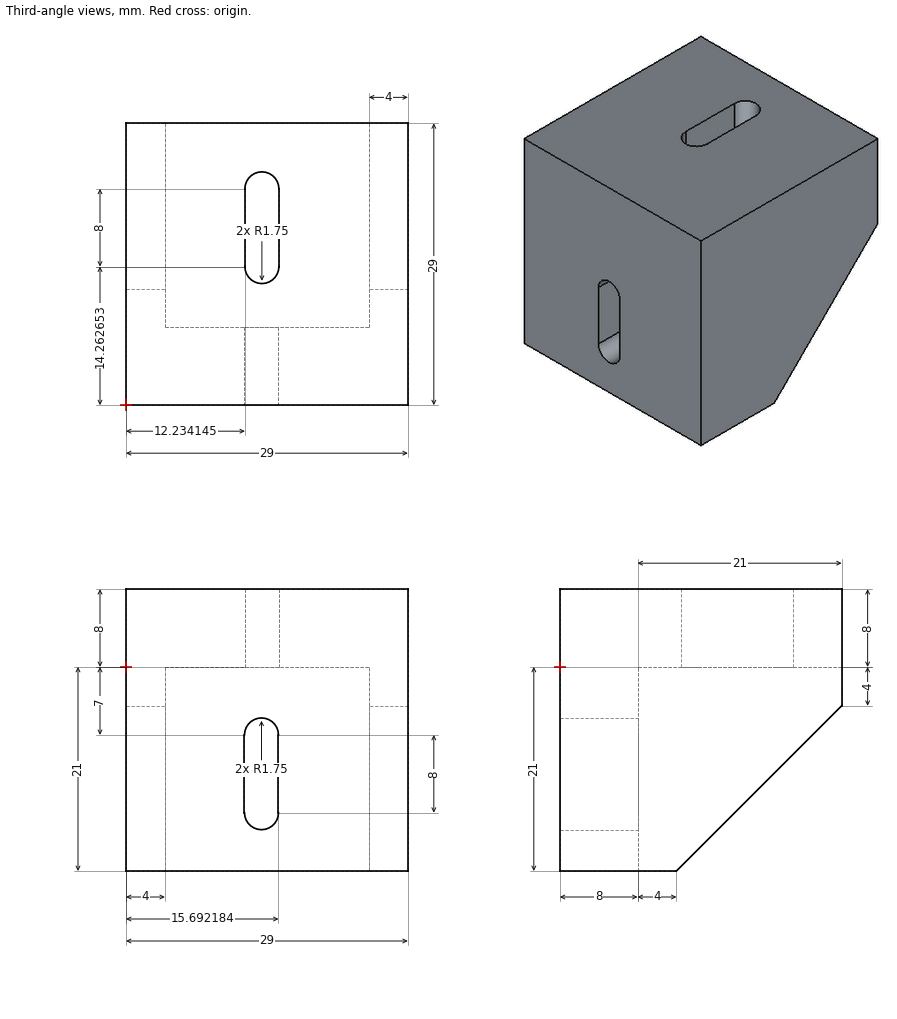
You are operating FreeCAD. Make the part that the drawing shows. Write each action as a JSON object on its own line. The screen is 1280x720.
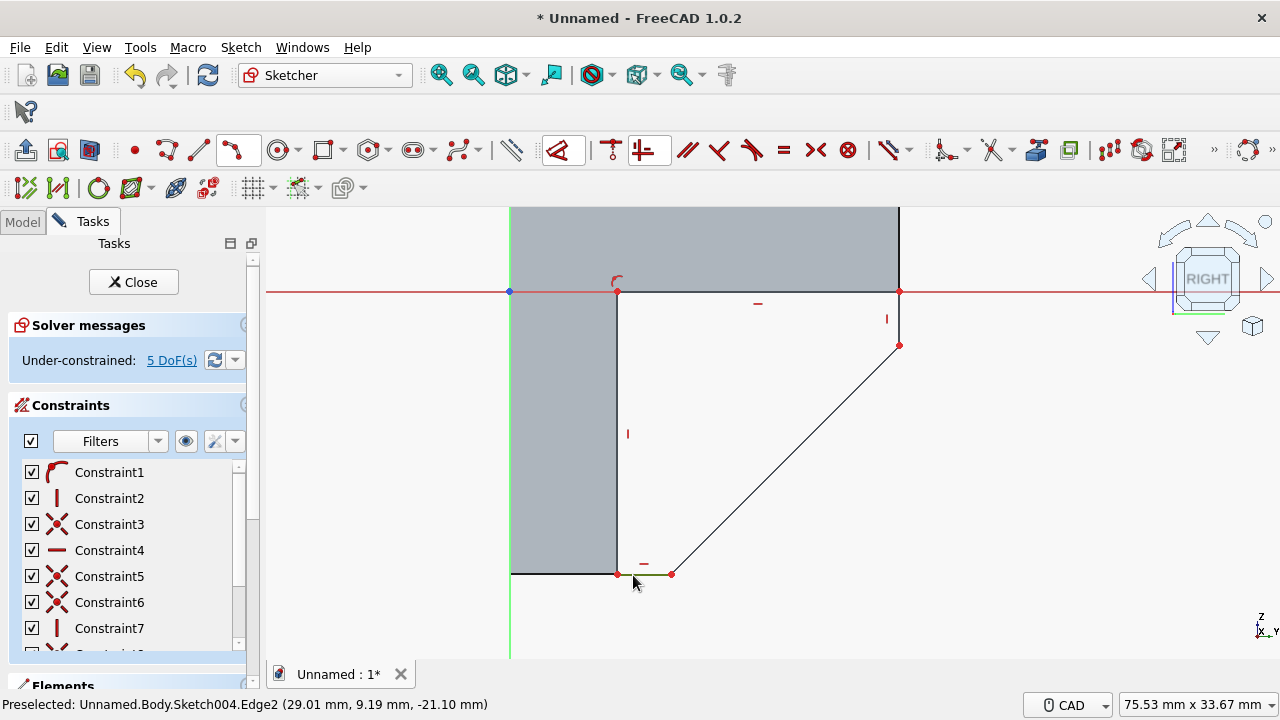
{"action": "left_click", "coordinate": [580, 150]}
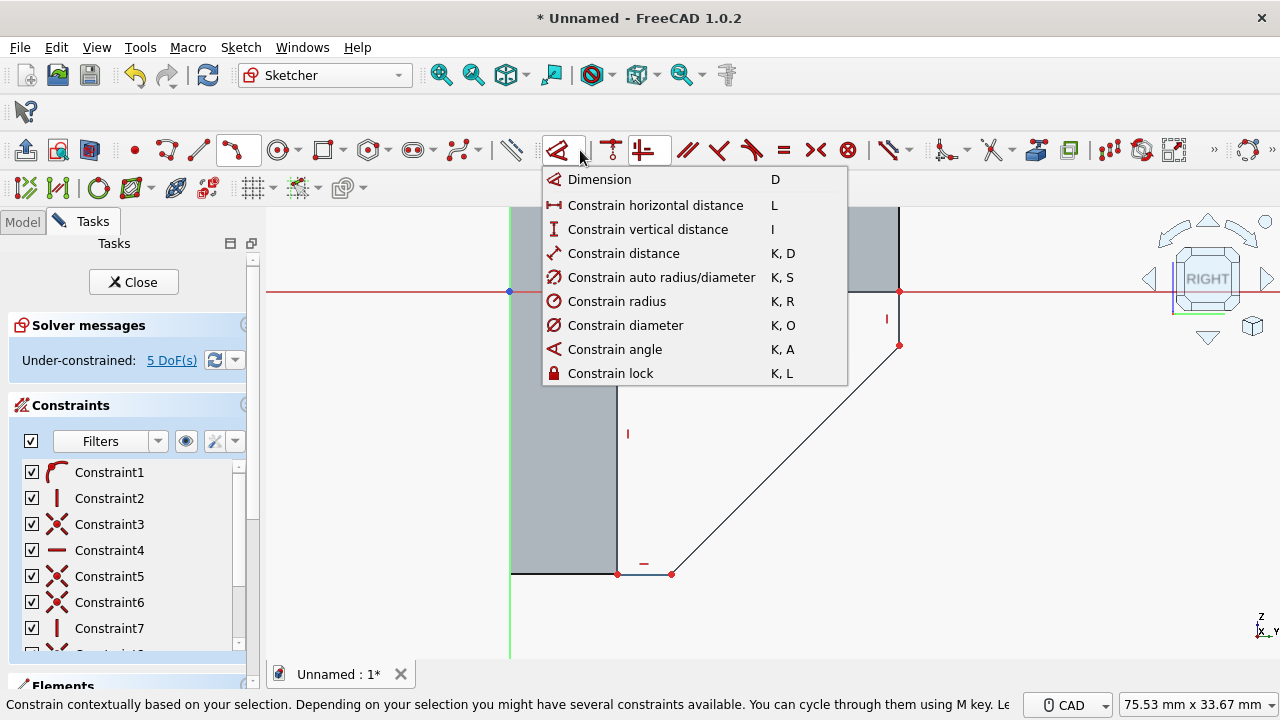
{"action": "left_click", "coordinate": [695, 205]}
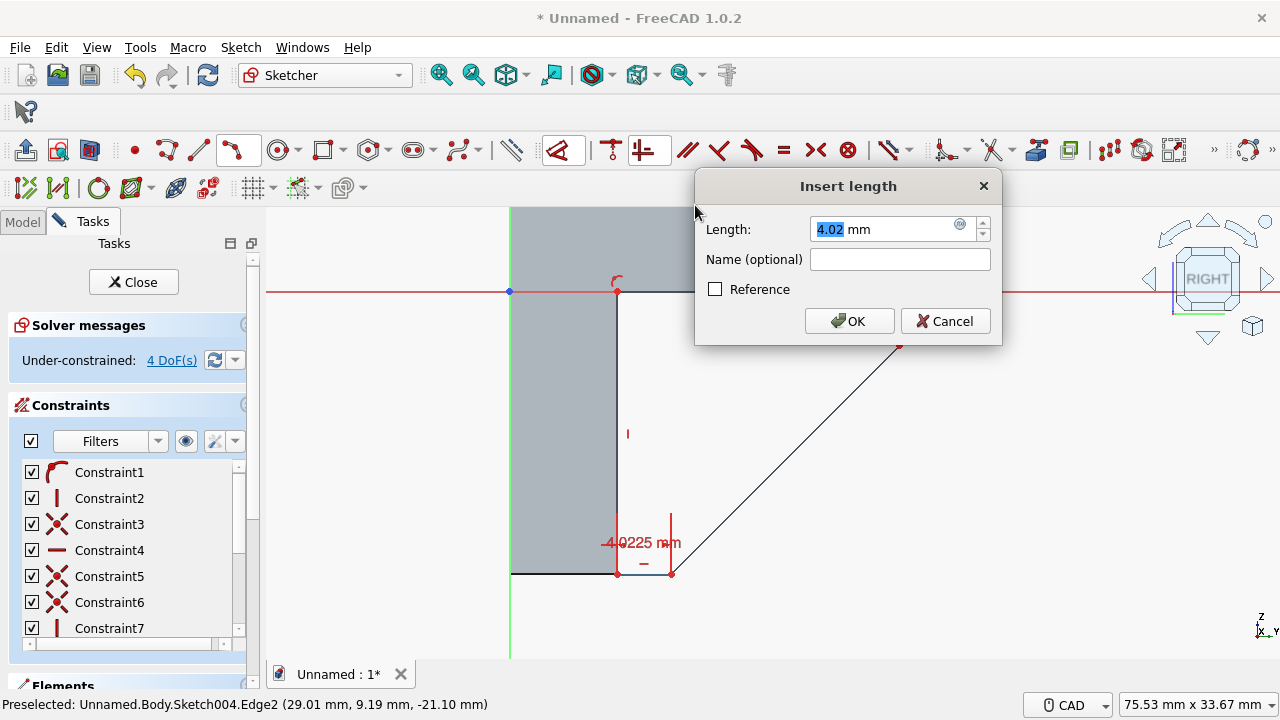
{"action": "type", "text": "4"}
{"action": "key", "text": "Return"}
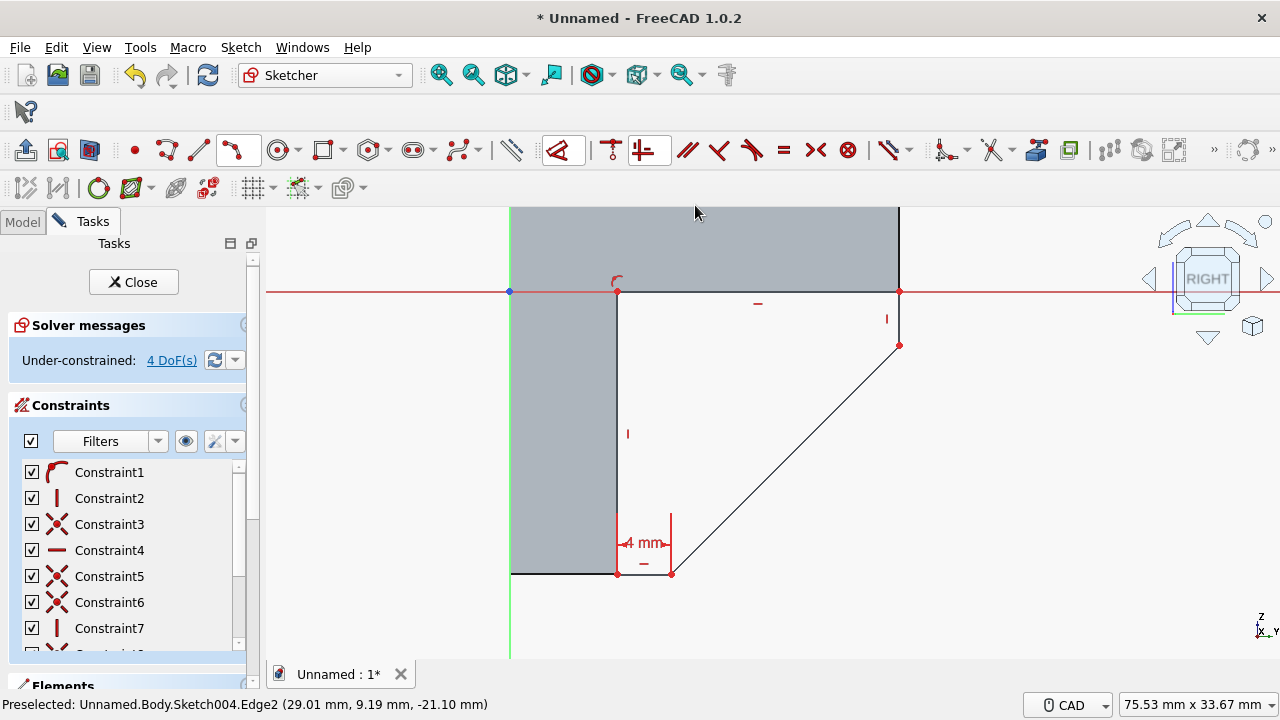
{"action": "left_click", "coordinate": [899, 330]}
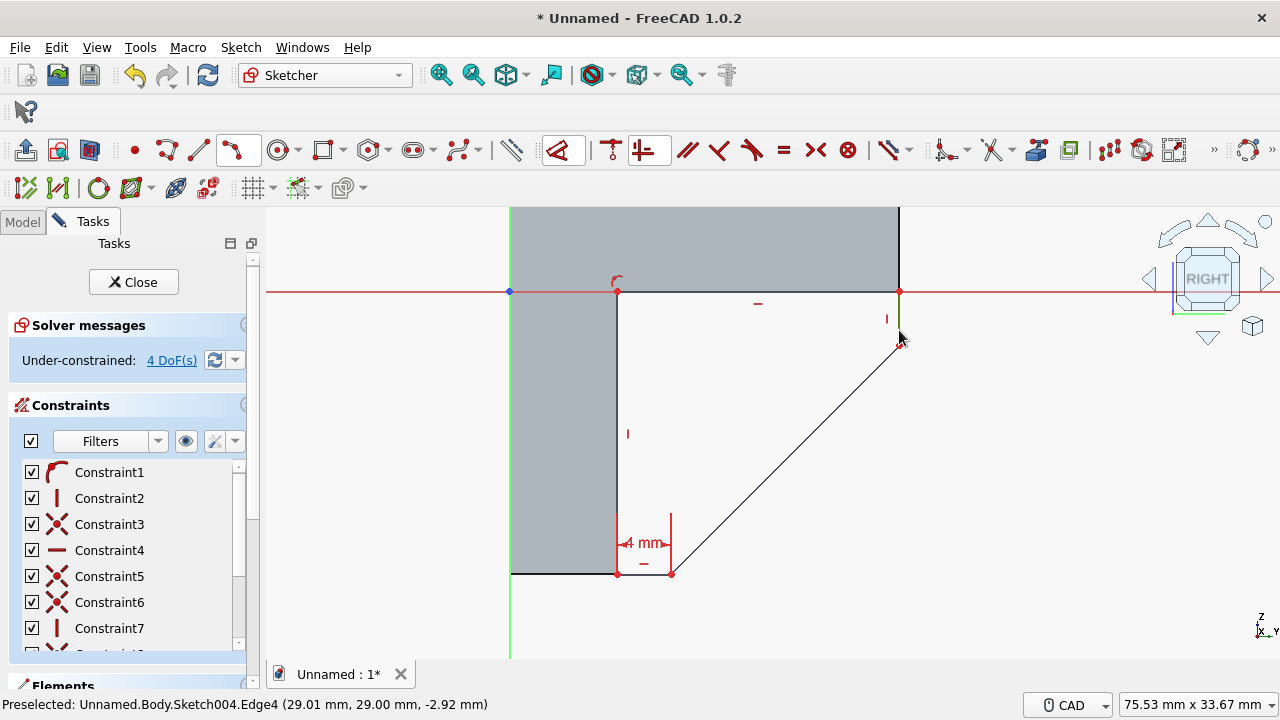
{"action": "key", "text": "i"}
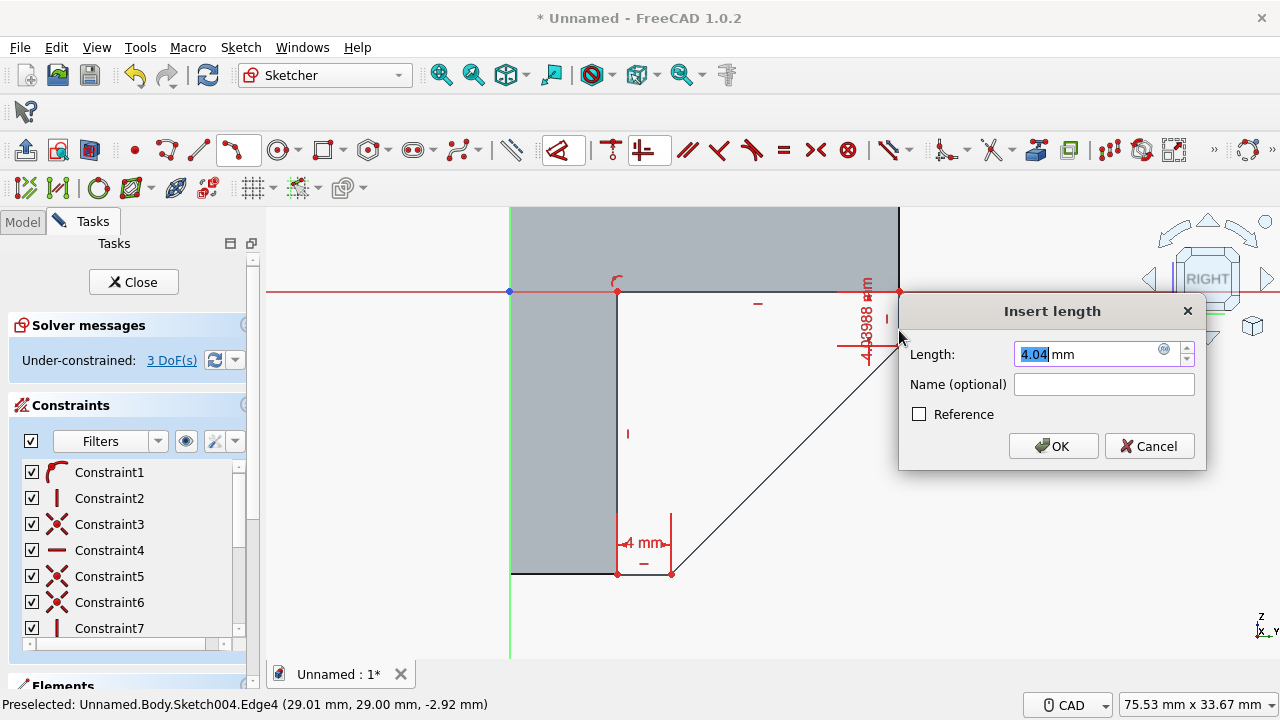
{"action": "type", "text": "4"}
{"action": "key", "text": "Return"}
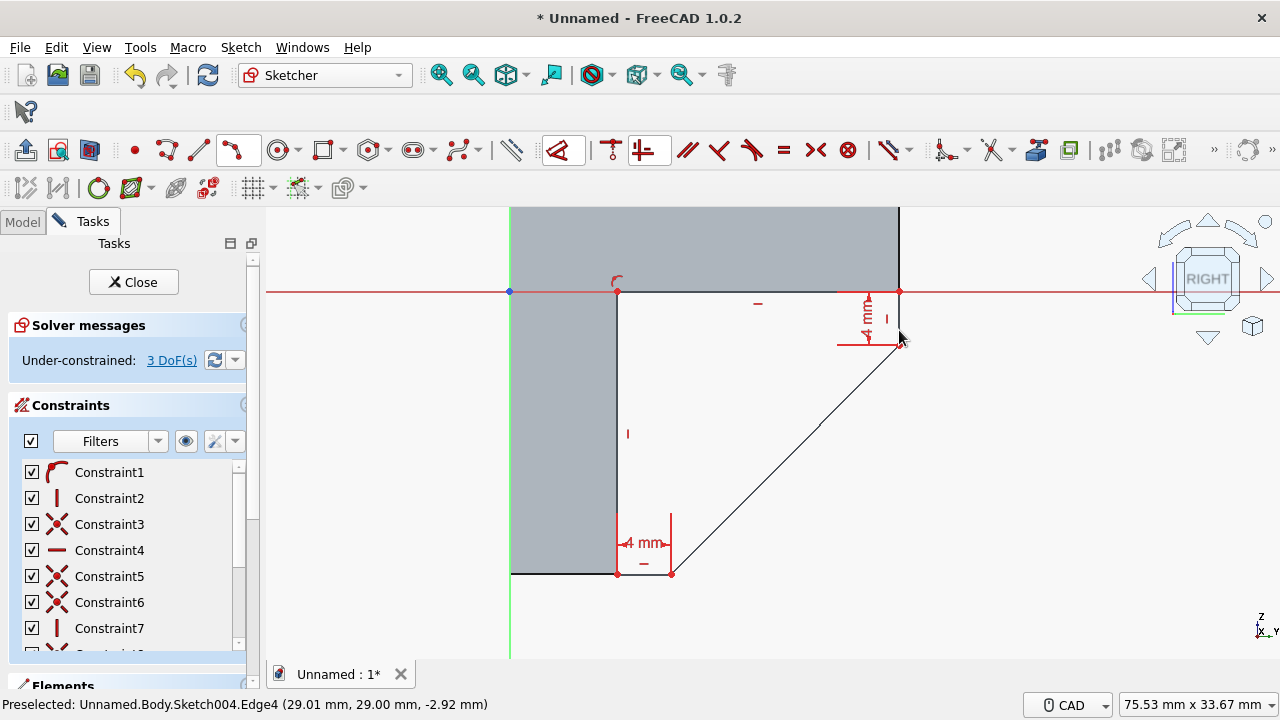
{"action": "left_click", "coordinate": [617, 377]}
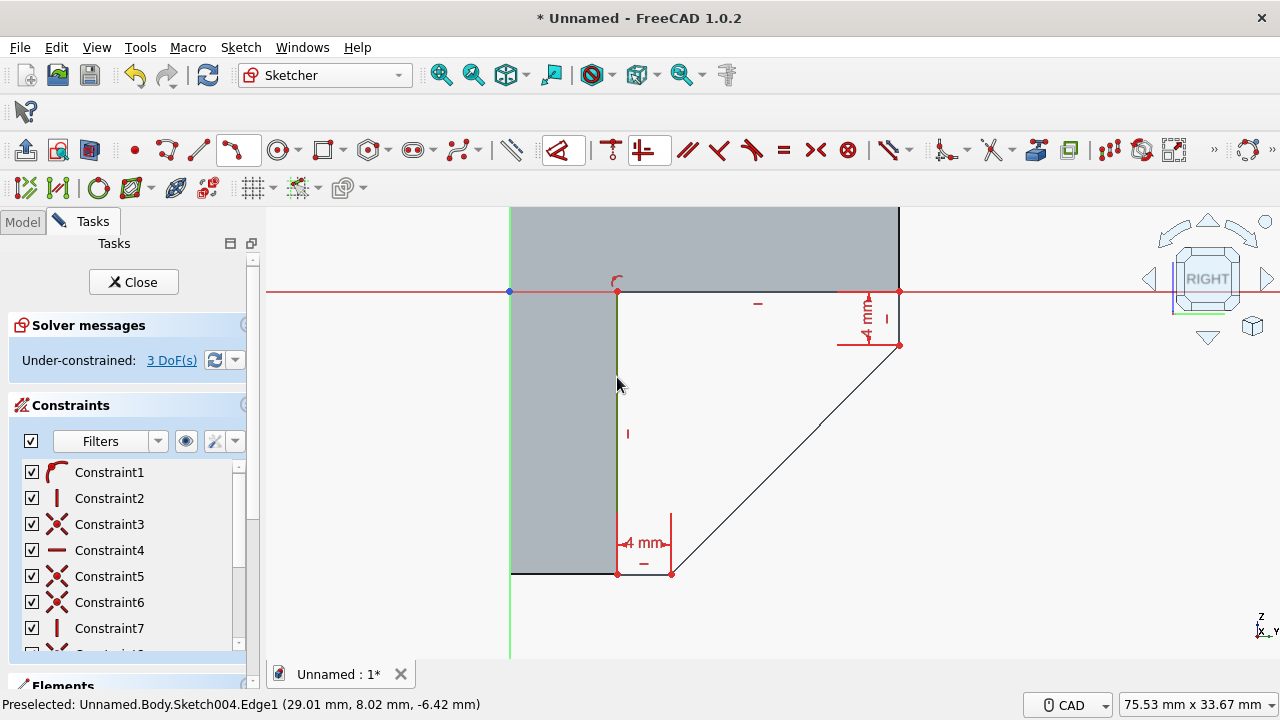
{"action": "left_click", "coordinate": [580, 150]}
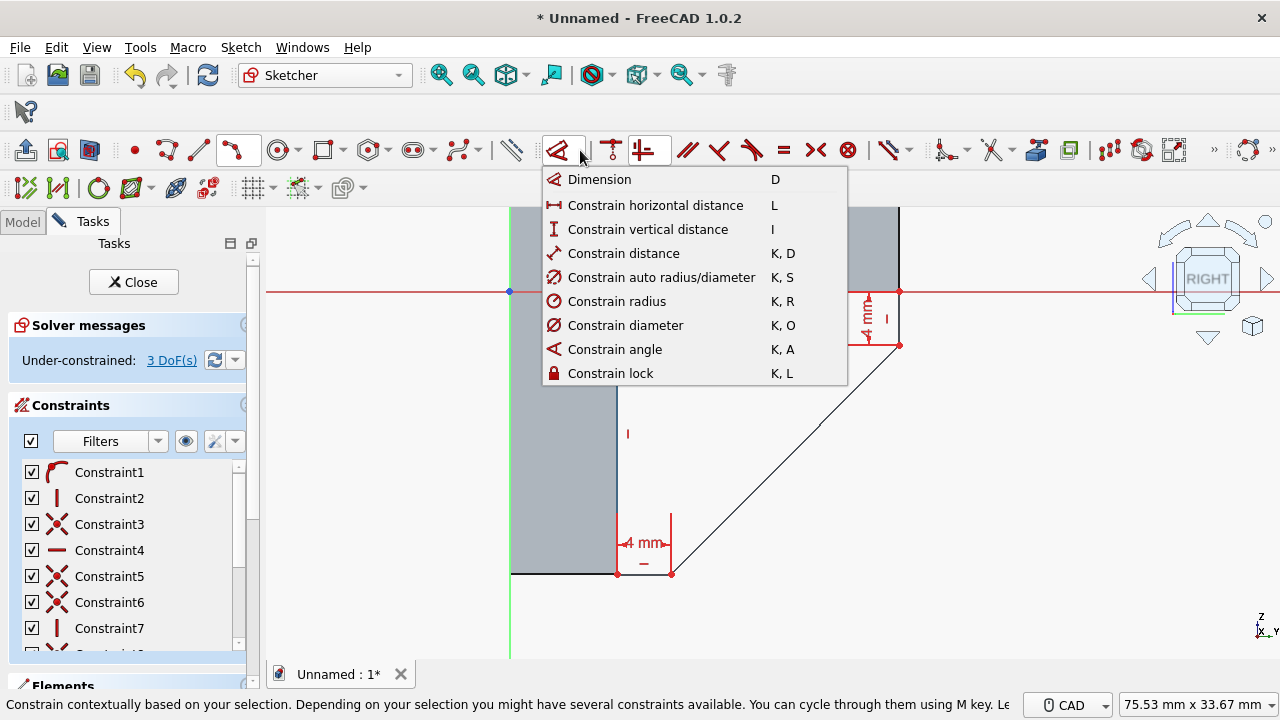
{"action": "left_click", "coordinate": [695, 229]}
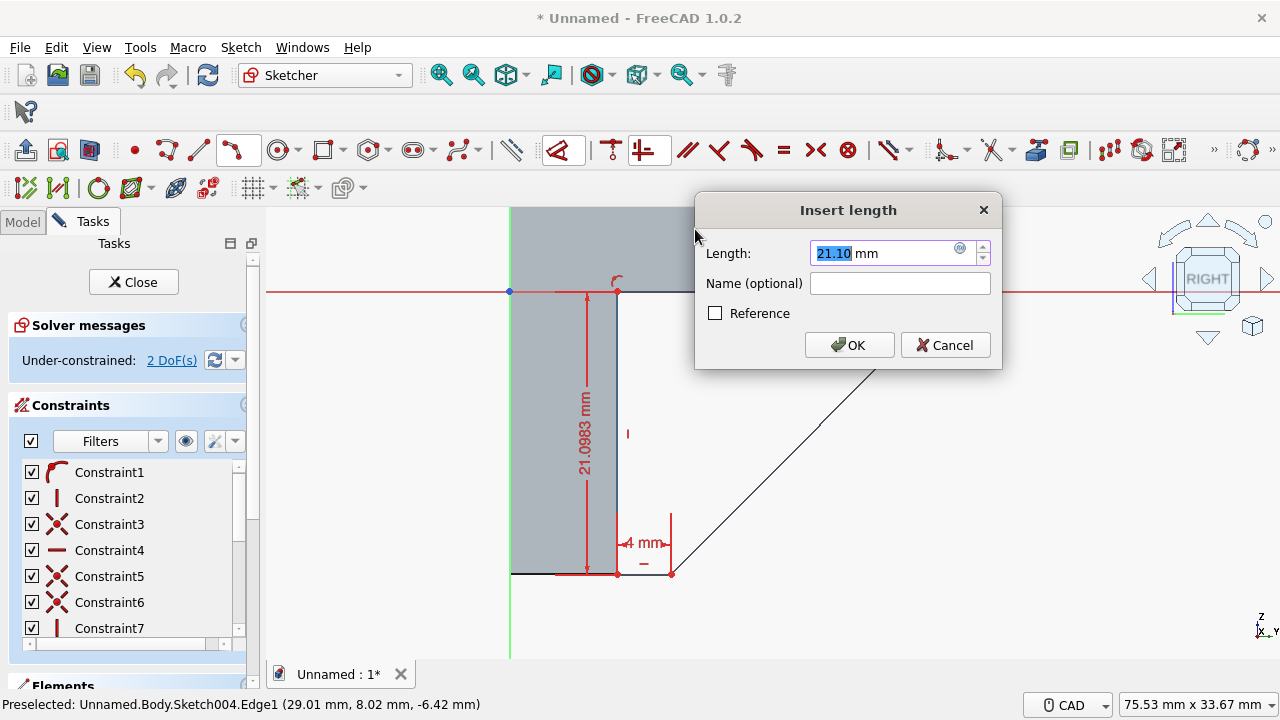
{"action": "type", "text": "21"}
{"action": "key", "text": "Return"}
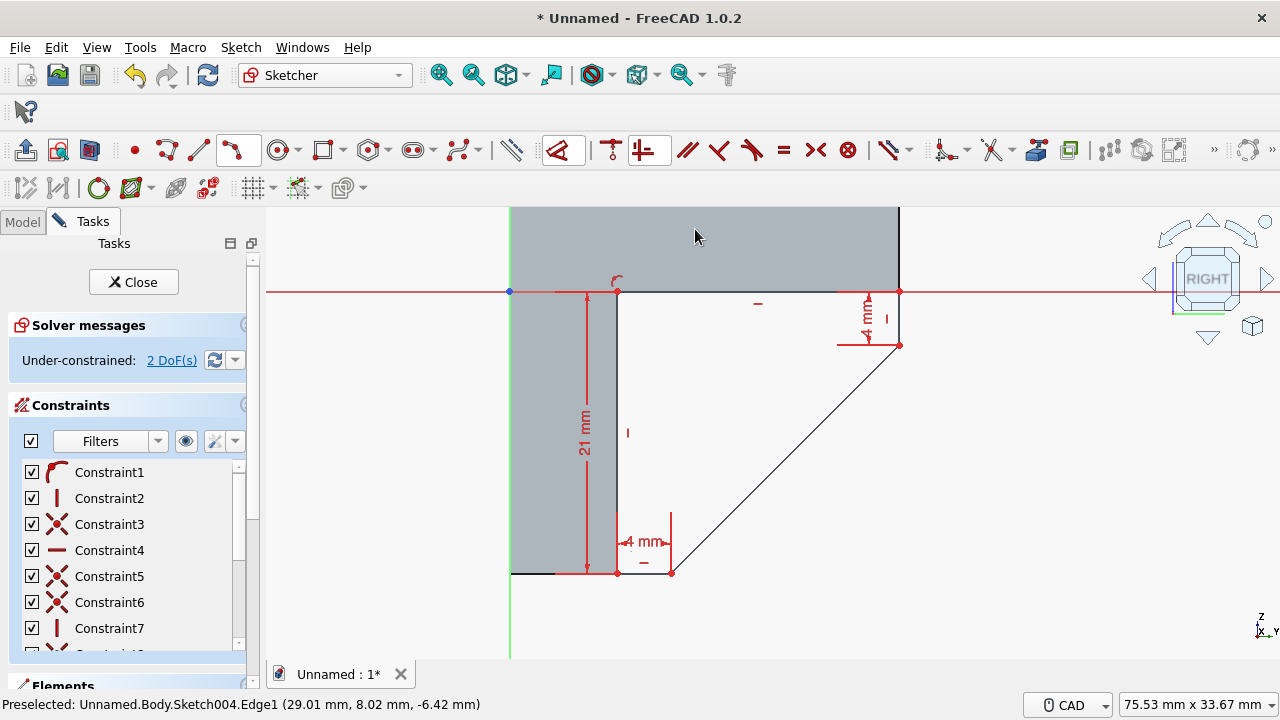
{"action": "left_click", "coordinate": [814, 292]}